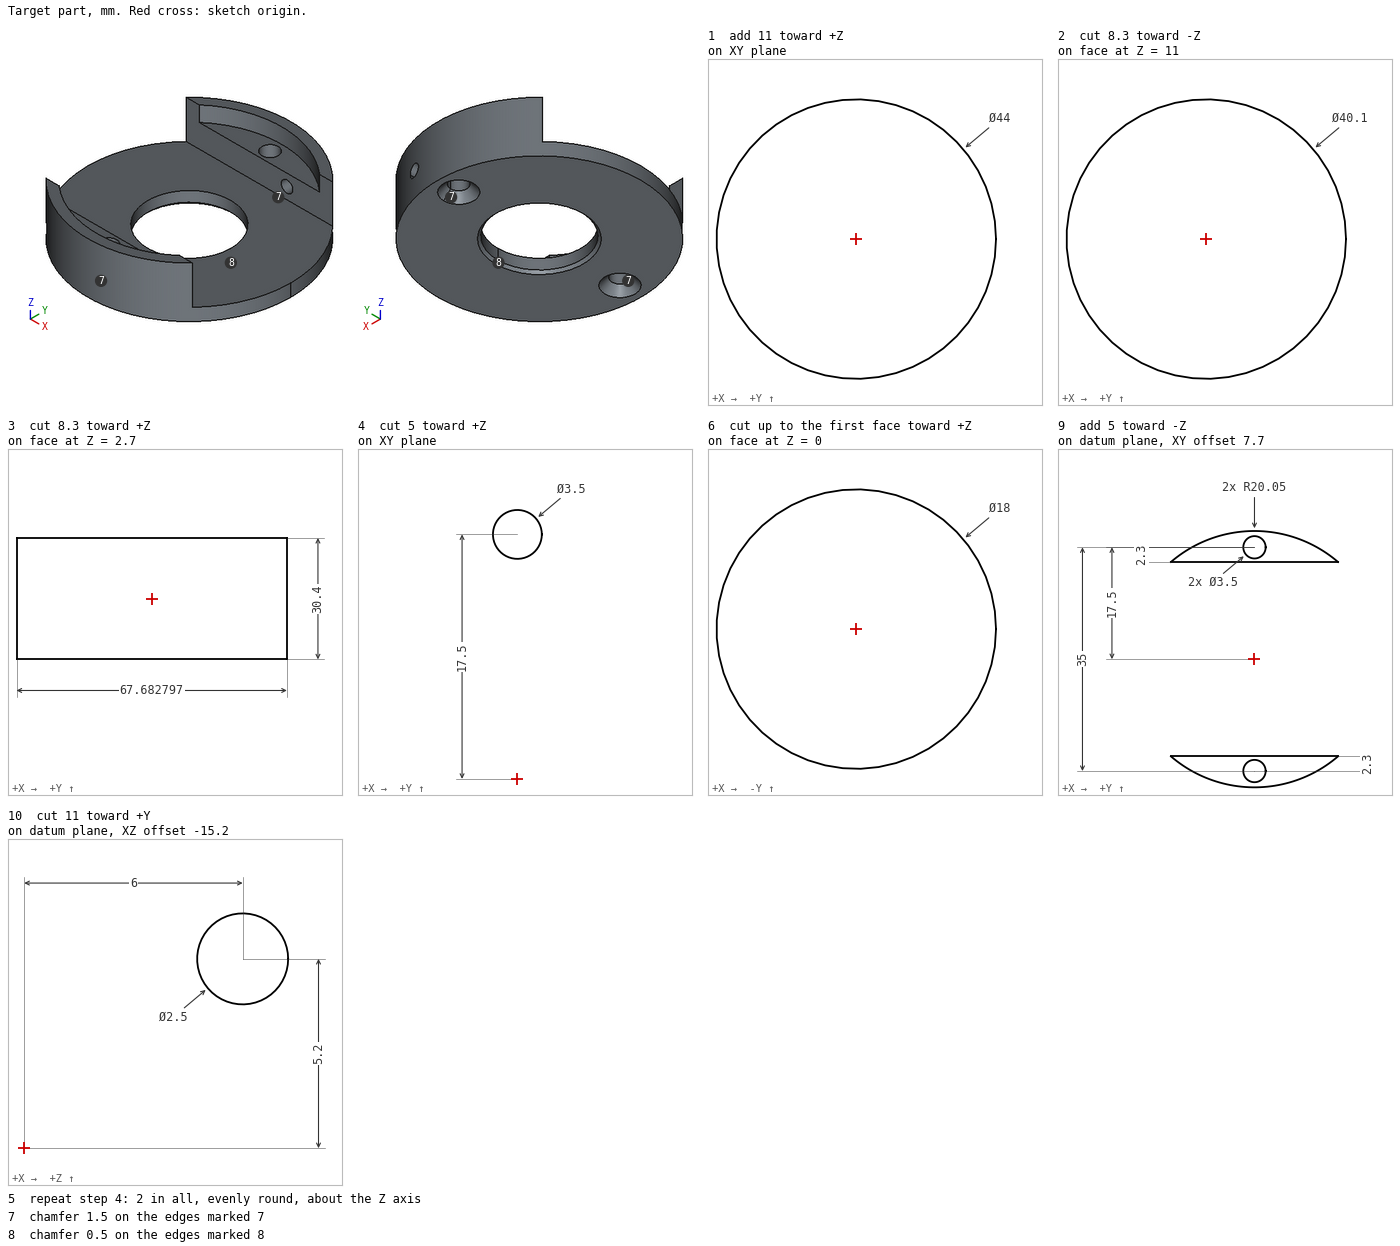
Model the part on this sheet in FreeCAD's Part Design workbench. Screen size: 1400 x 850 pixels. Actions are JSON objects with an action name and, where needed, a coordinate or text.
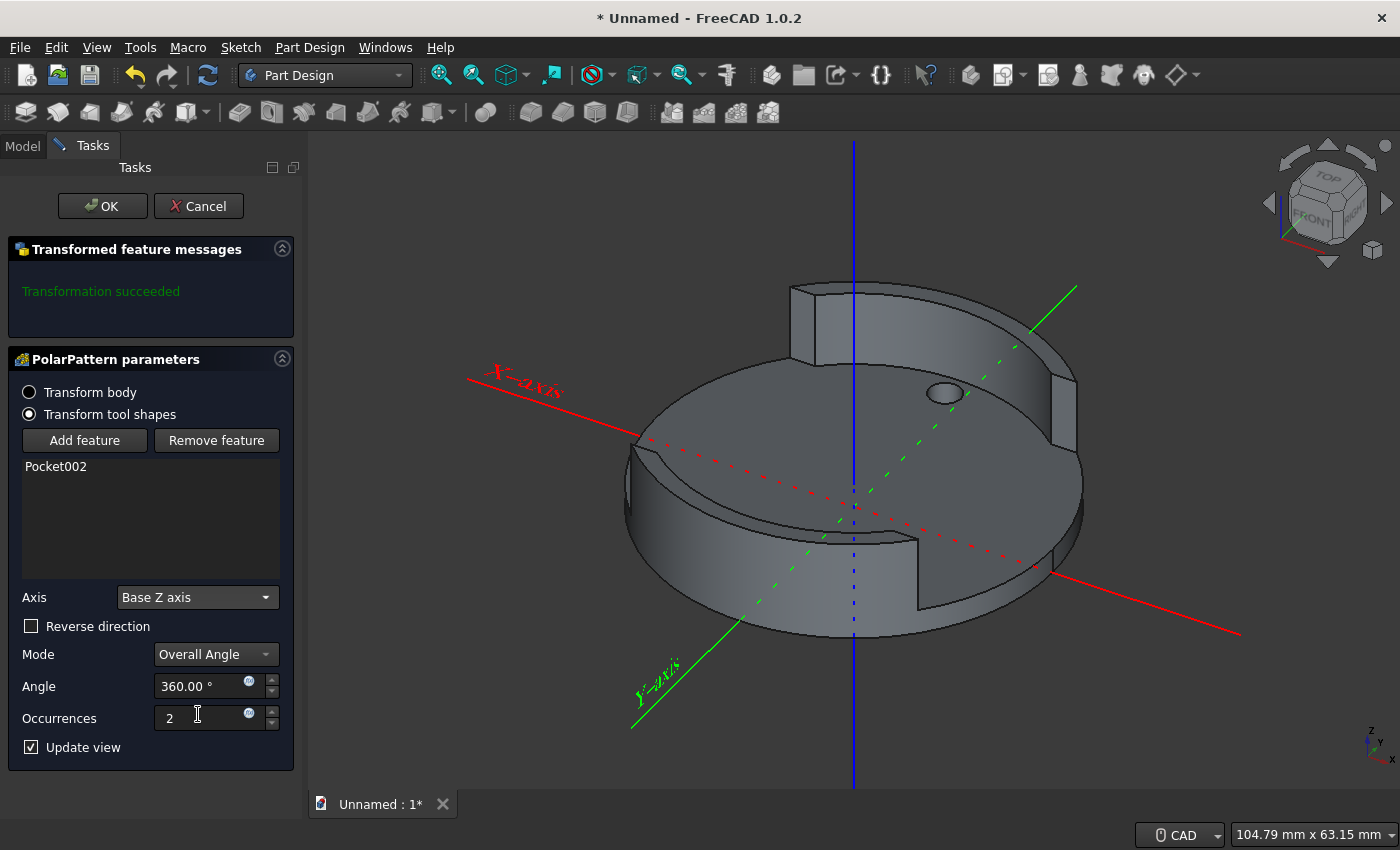
{"action": "triple_click", "coordinate": [209, 718]}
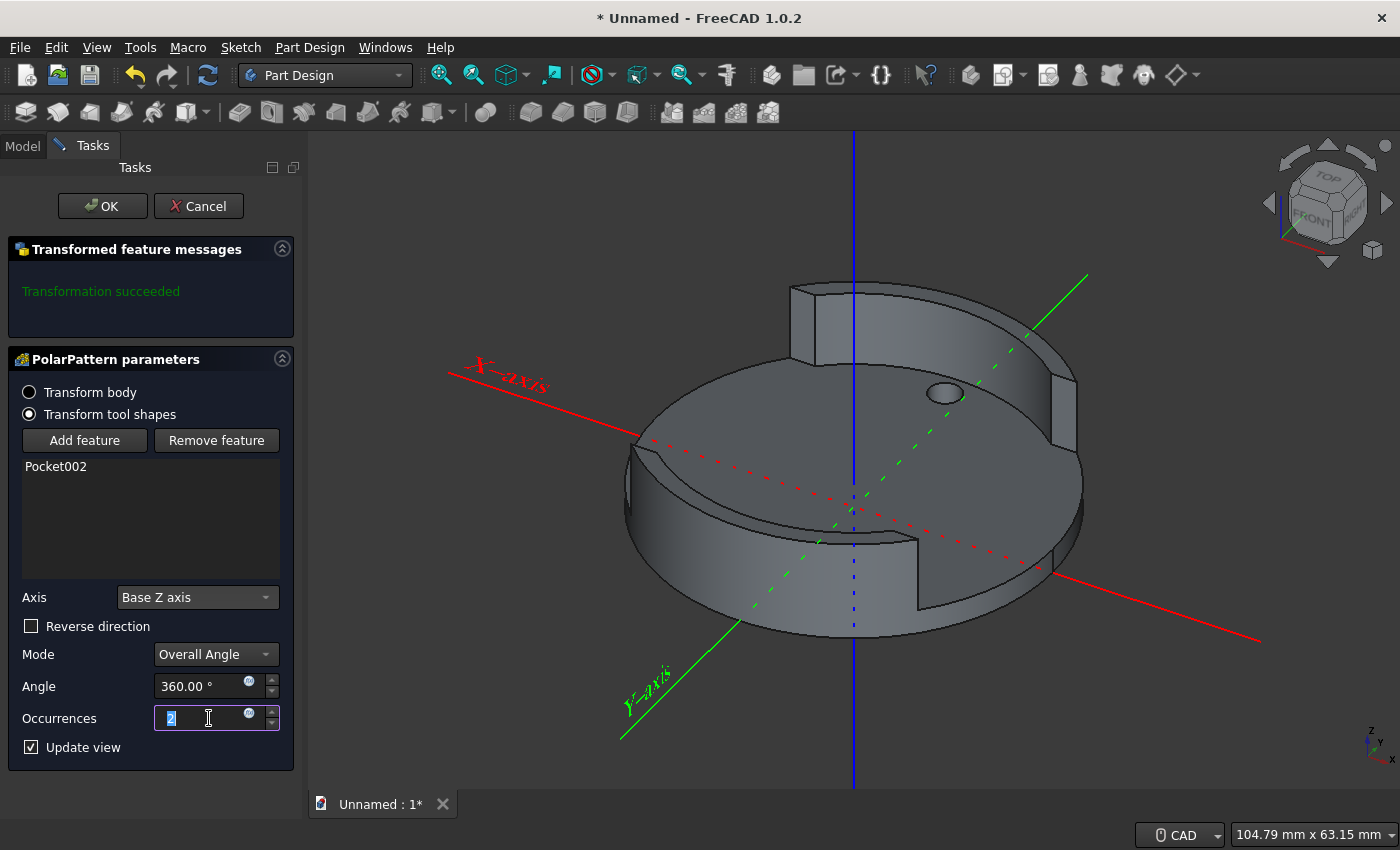
{"action": "type", "text": "2"}
{"action": "key", "text": "Tab"}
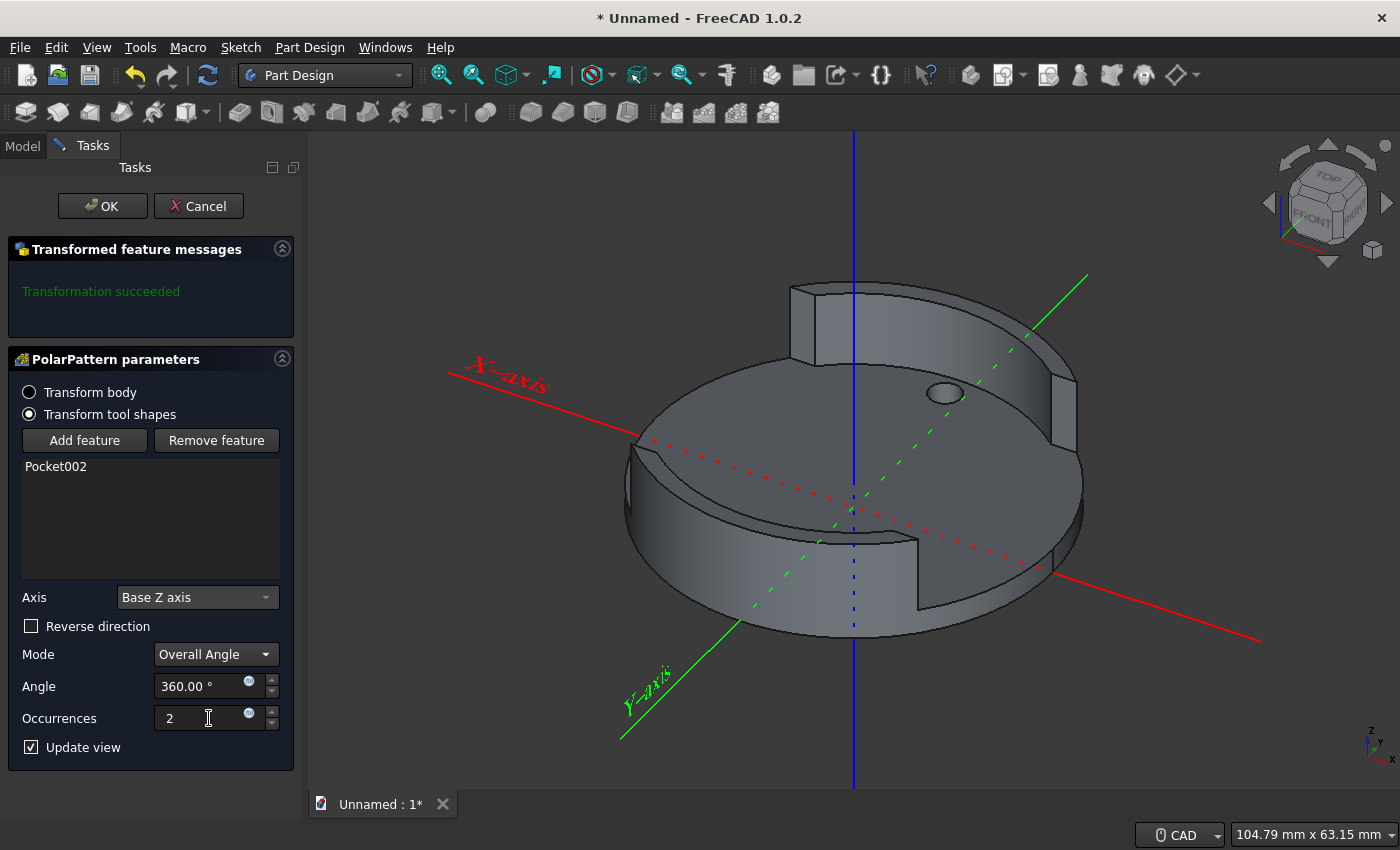
{"action": "left_click", "coordinate": [103, 206]}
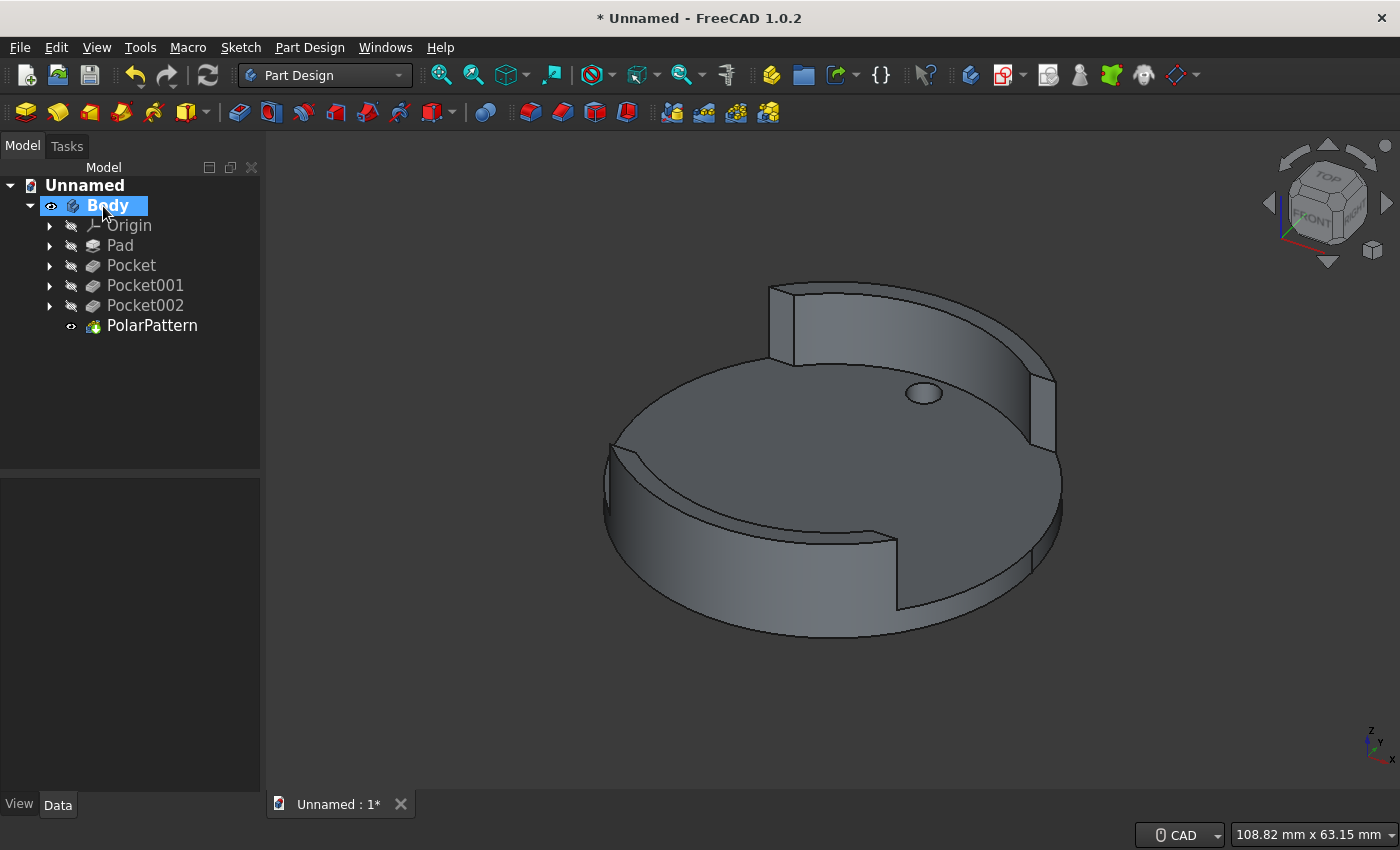
{"action": "key", "text": "5"}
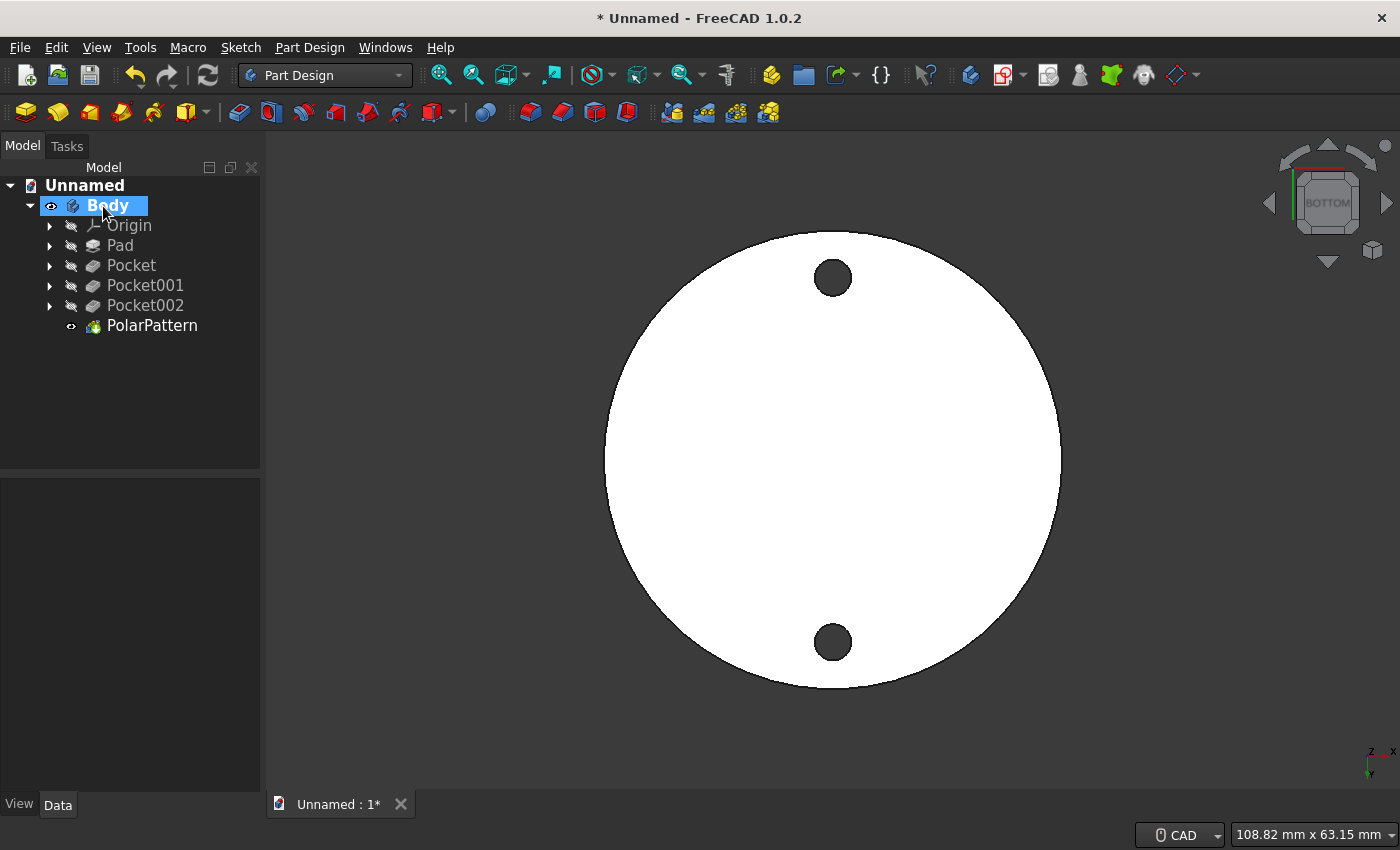
{"action": "left_click", "coordinate": [833, 459]}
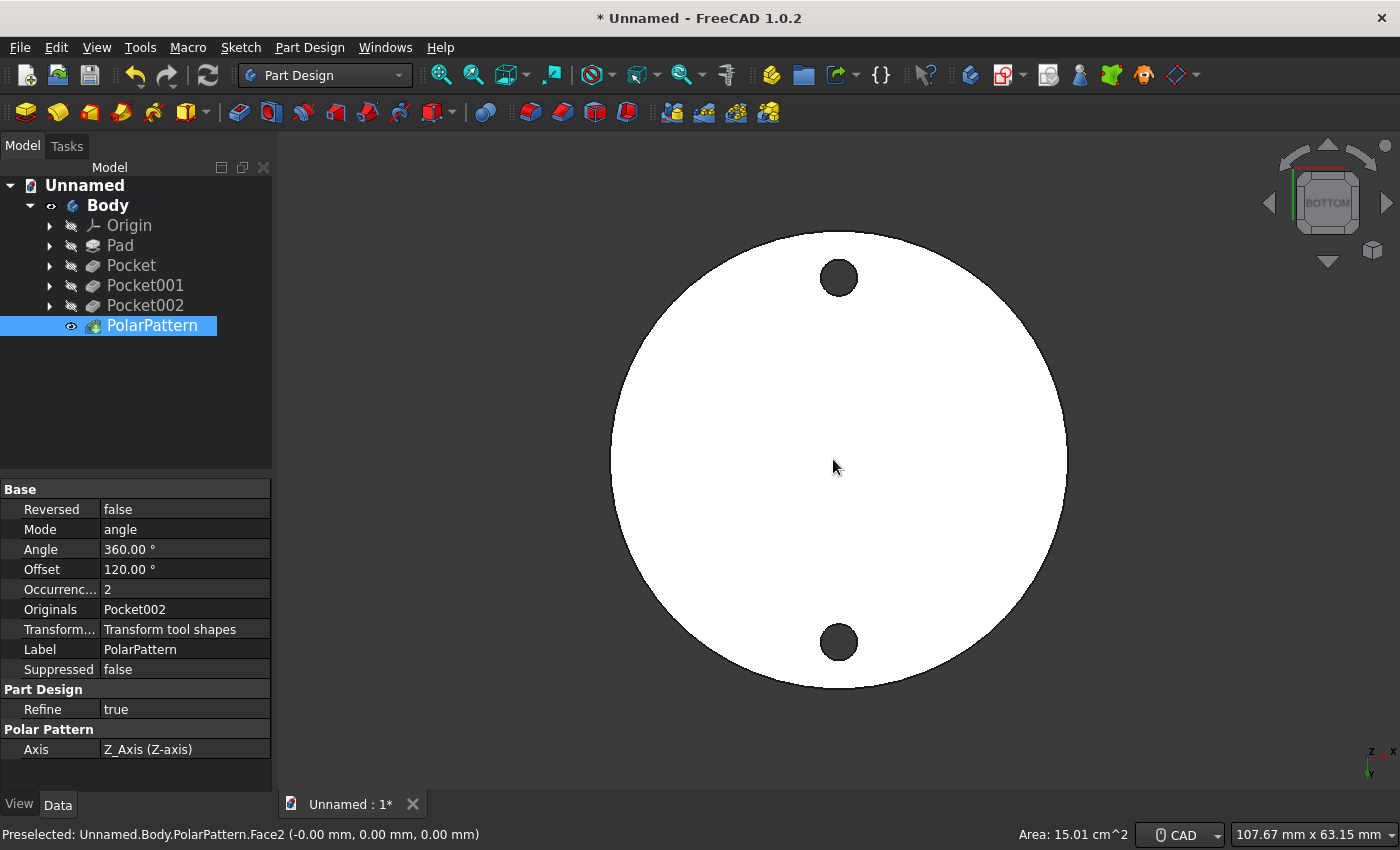
{"action": "left_click", "coordinate": [1004, 76]}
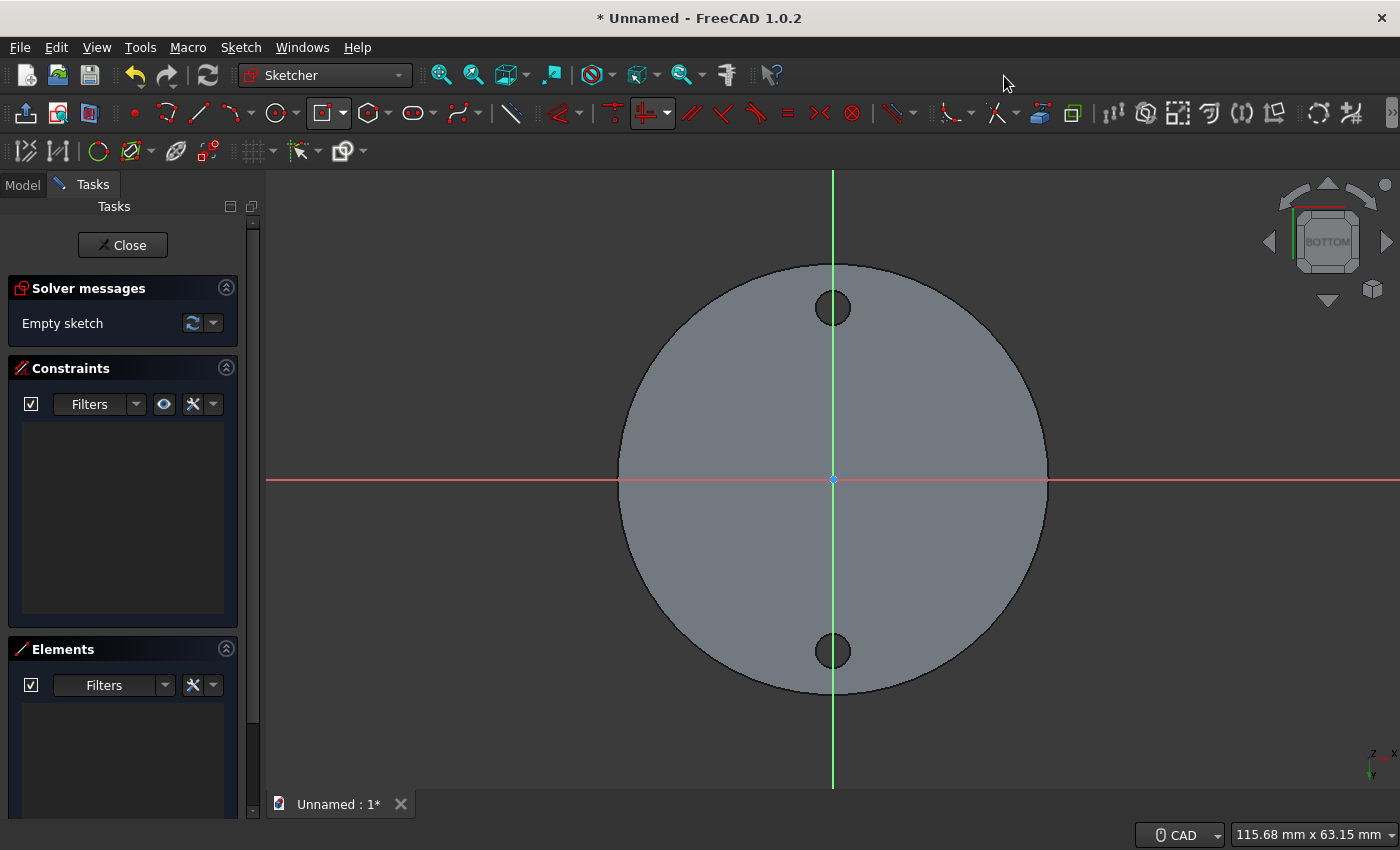
{"action": "scroll", "coordinate": [889, 480], "scroll_direction": "up", "scroll_amount": 4}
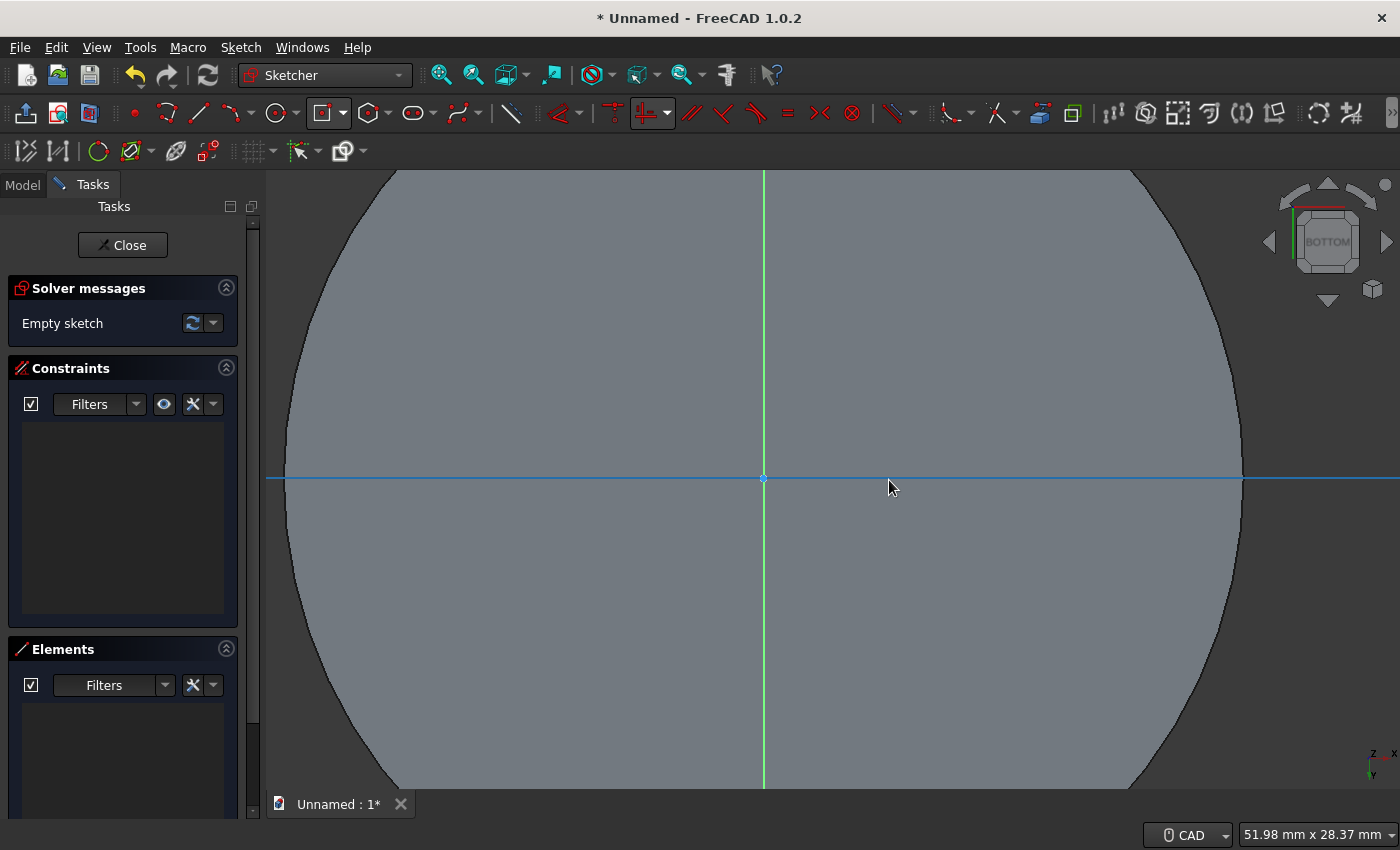
{"action": "key", "text": "g c"}